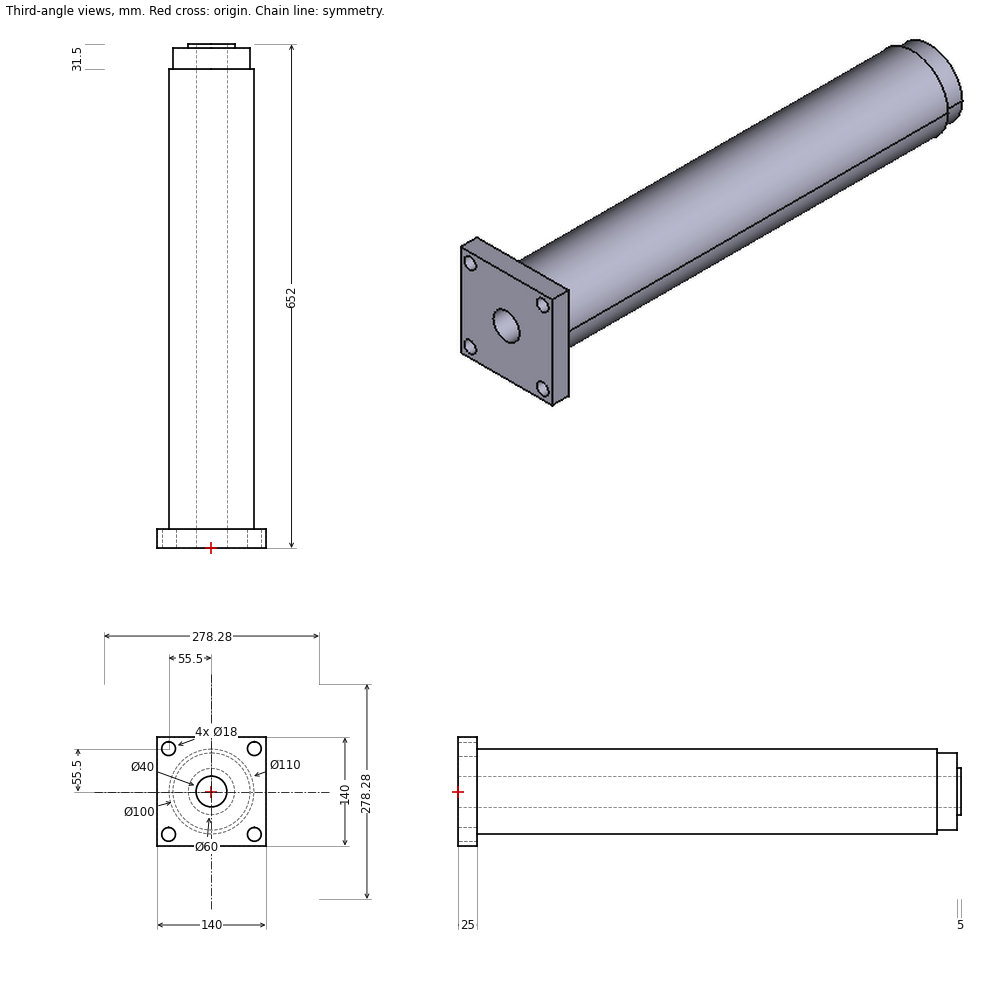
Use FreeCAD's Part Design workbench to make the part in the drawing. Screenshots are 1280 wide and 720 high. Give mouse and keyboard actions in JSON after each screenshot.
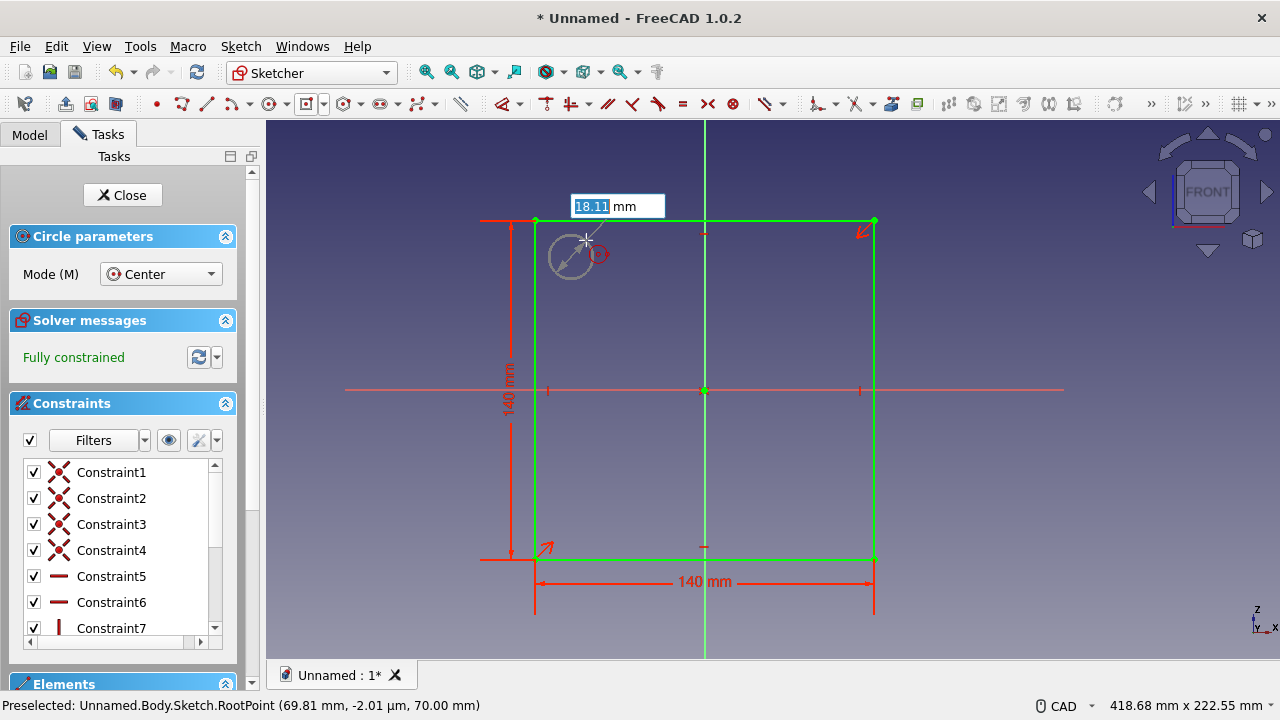
{"action": "type", "text": "18"}
{"action": "key", "text": "Return"}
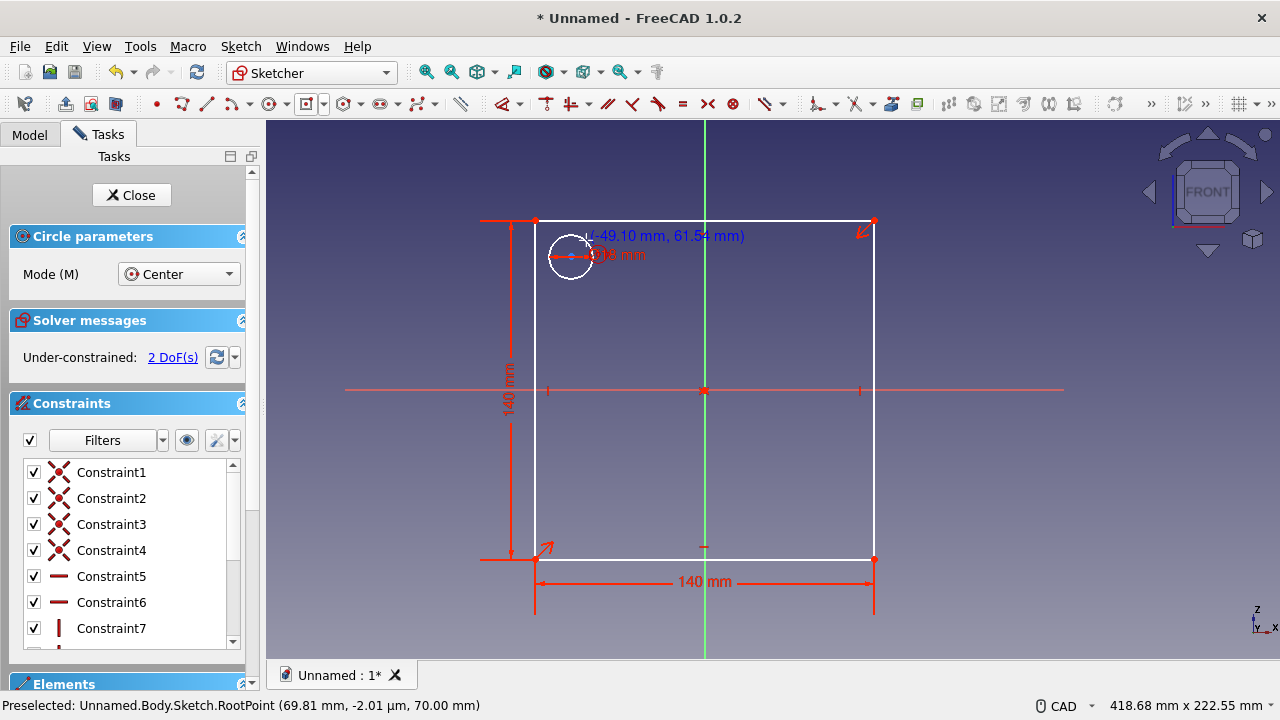
{"action": "left_click", "coordinate": [839, 256]}
{"action": "mouse_move", "coordinate": [855, 240]}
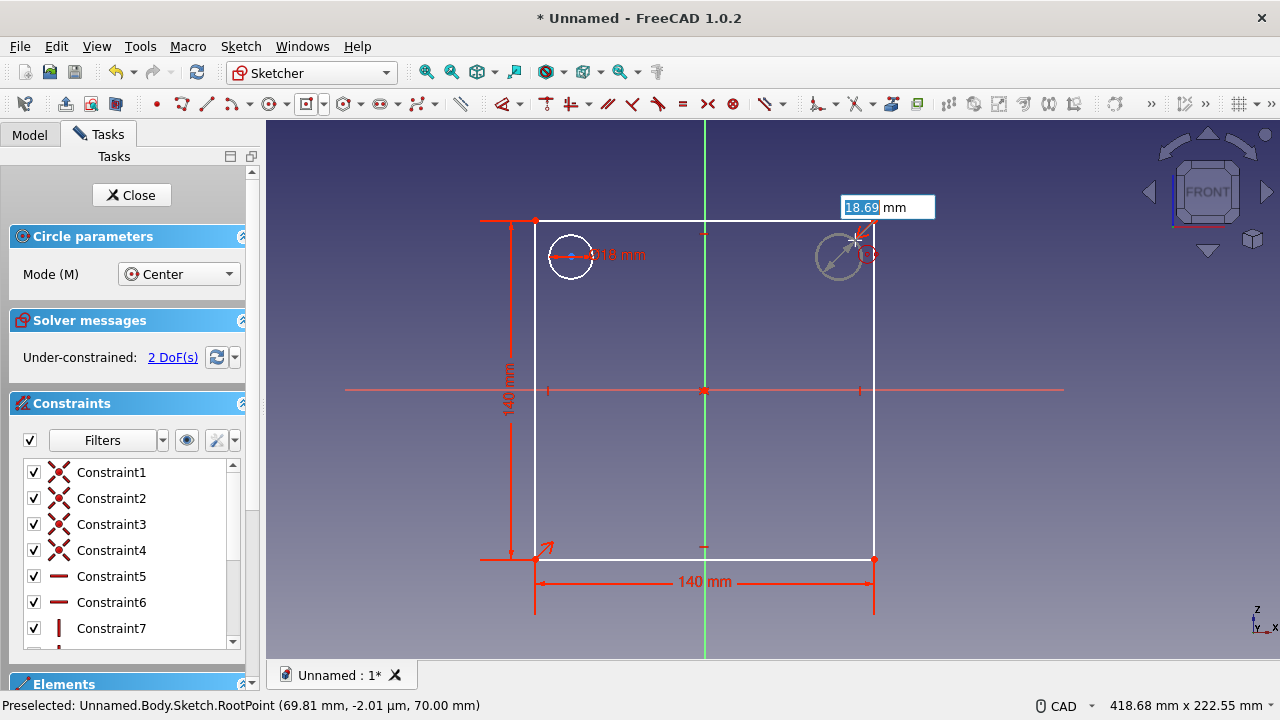
{"action": "type", "text": "18"}
{"action": "key", "text": "Return"}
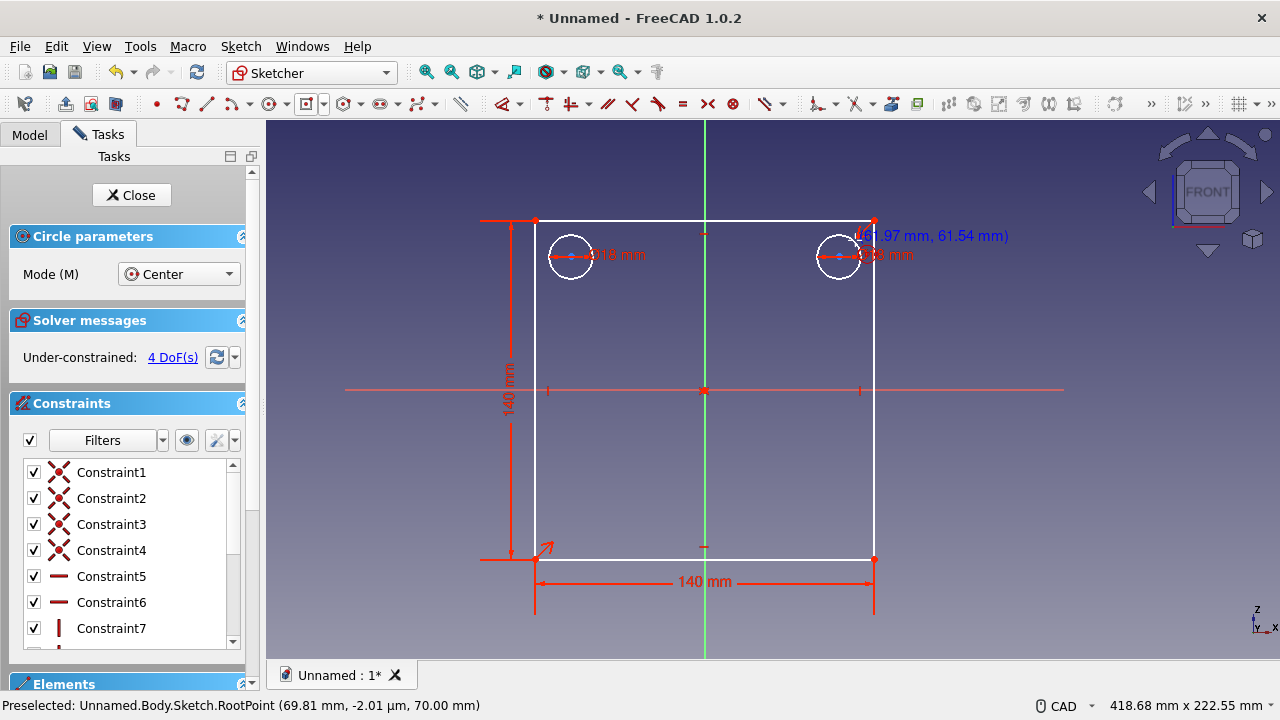
{"action": "left_click", "coordinate": [571, 524]}
{"action": "mouse_move", "coordinate": [586, 509]}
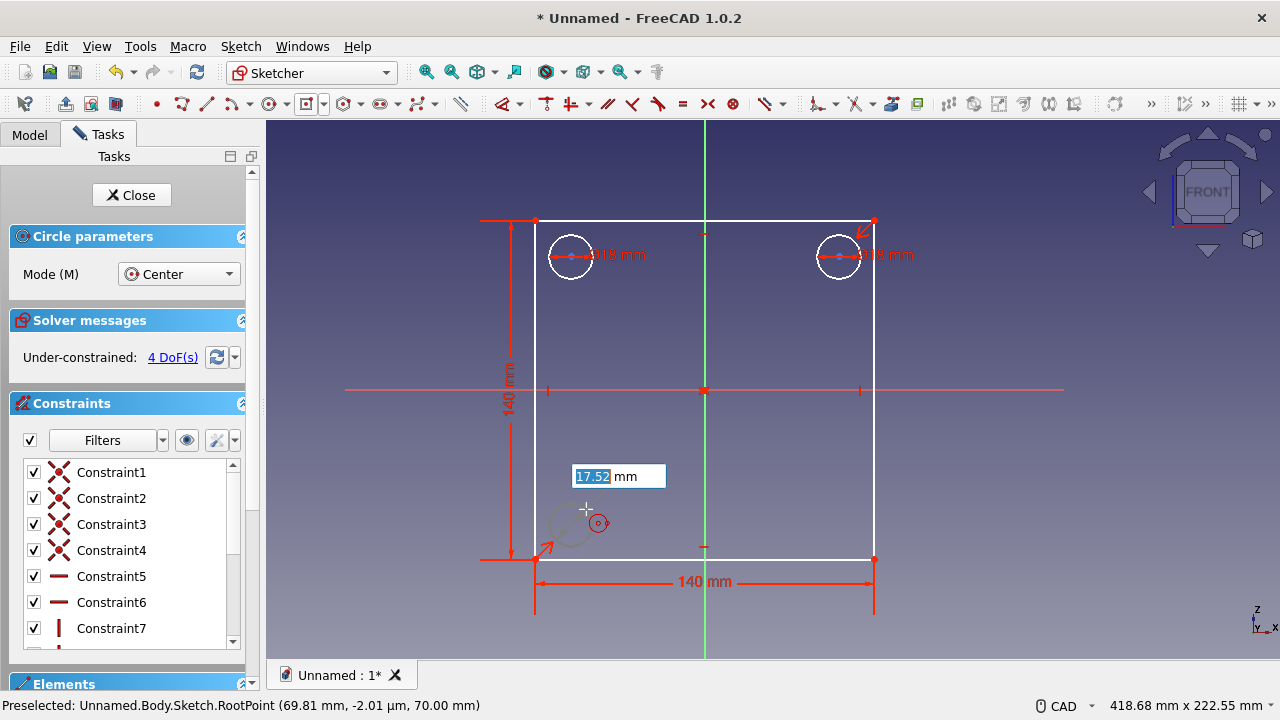
{"action": "type", "text": "18"}
{"action": "key", "text": "Return"}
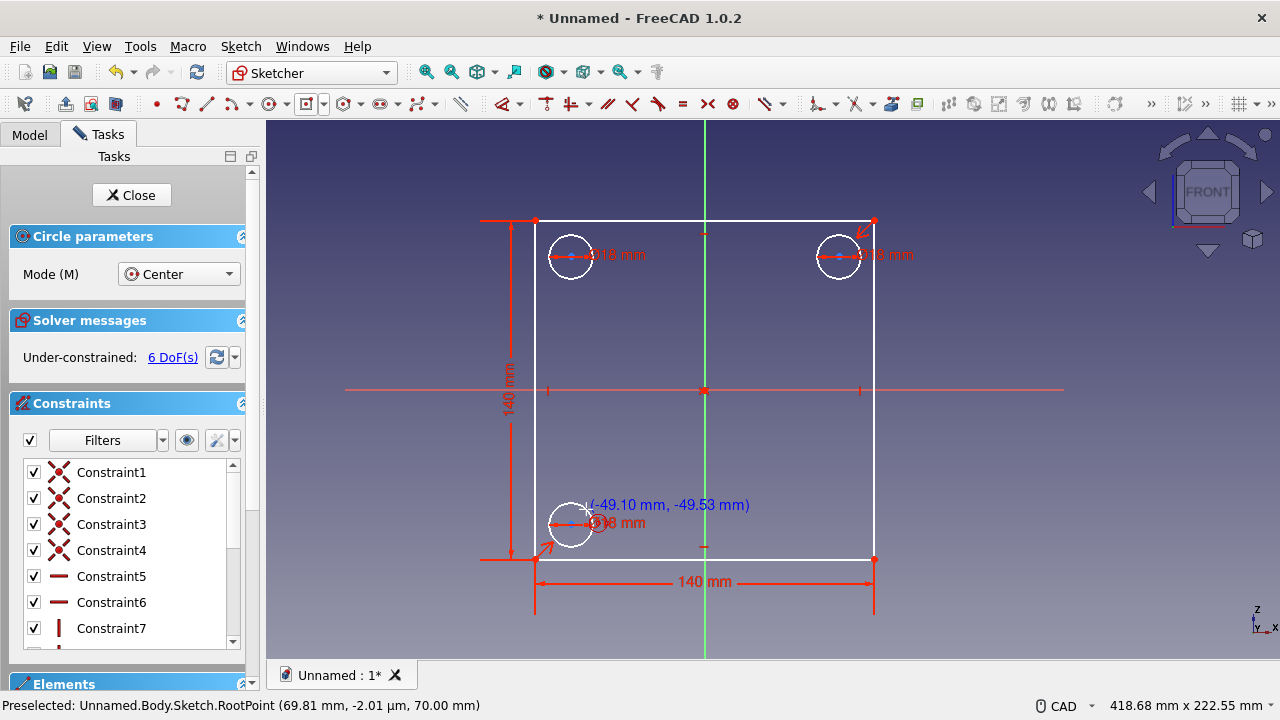
{"action": "left_click", "coordinate": [839, 524]}
{"action": "mouse_move", "coordinate": [855, 509]}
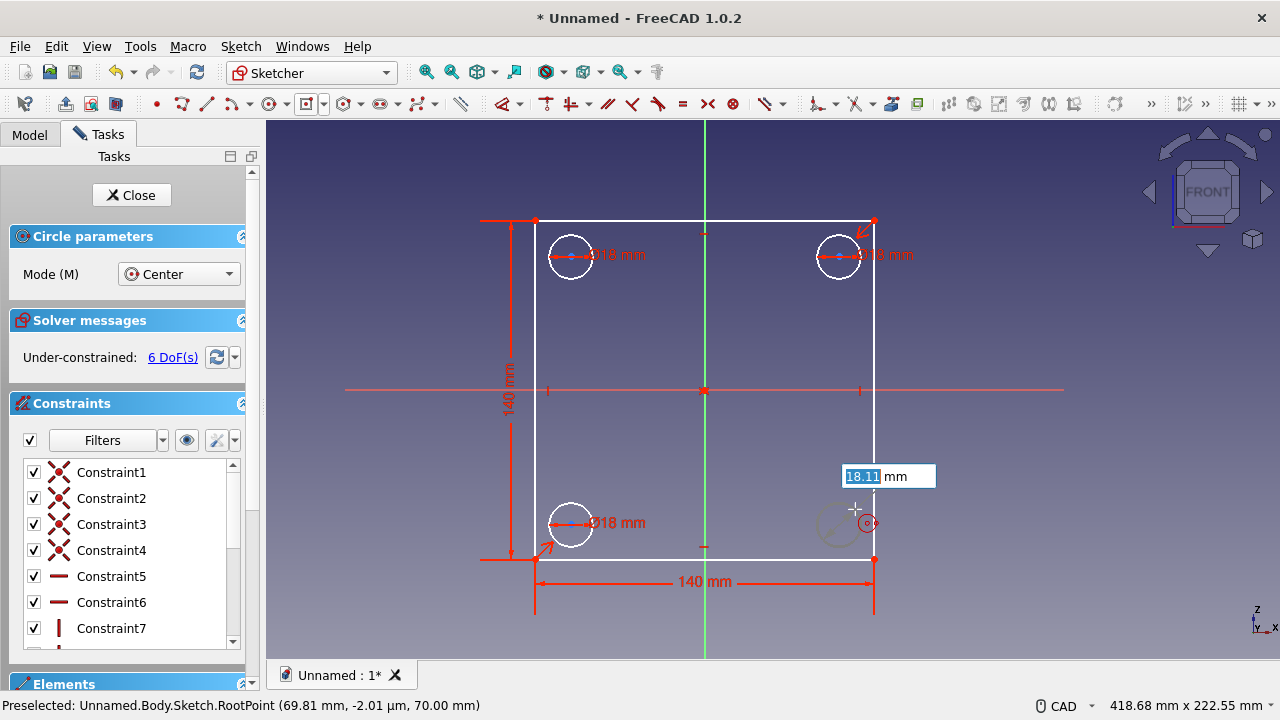
{"action": "type", "text": "18"}
{"action": "key", "text": "Return"}
{"action": "key", "text": "Escape"}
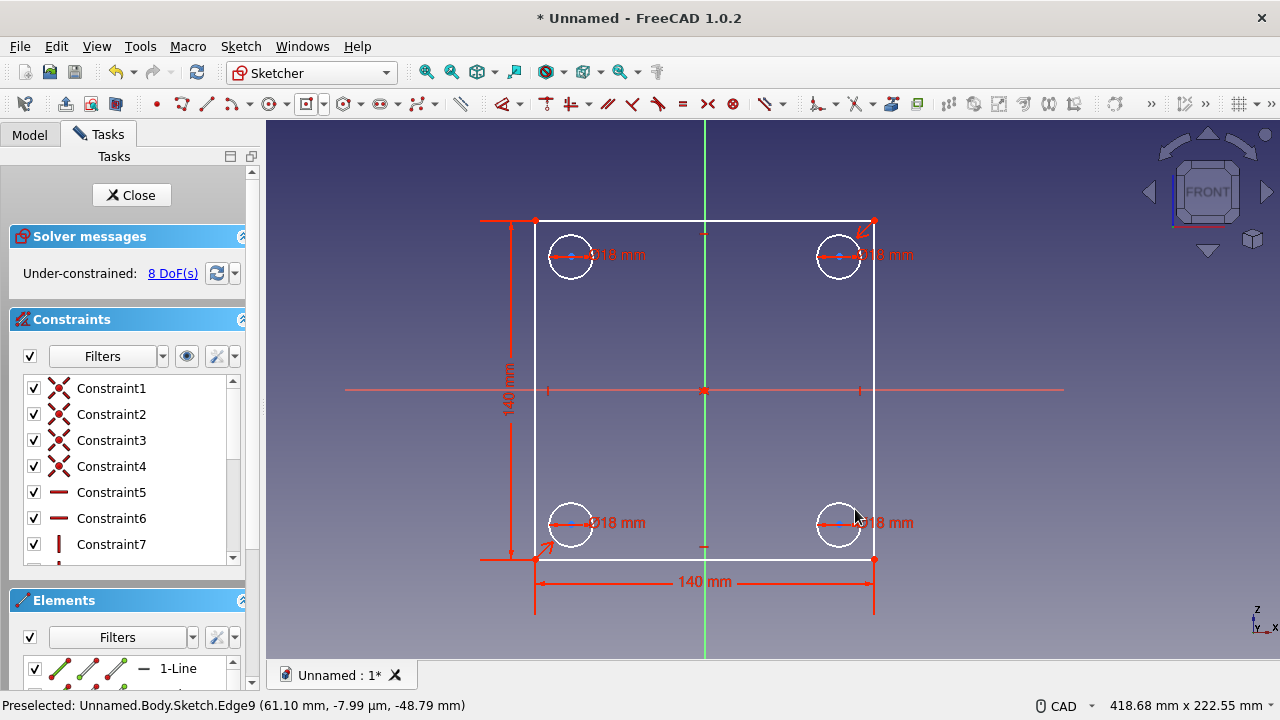
{"action": "left_click", "coordinate": [571, 257]}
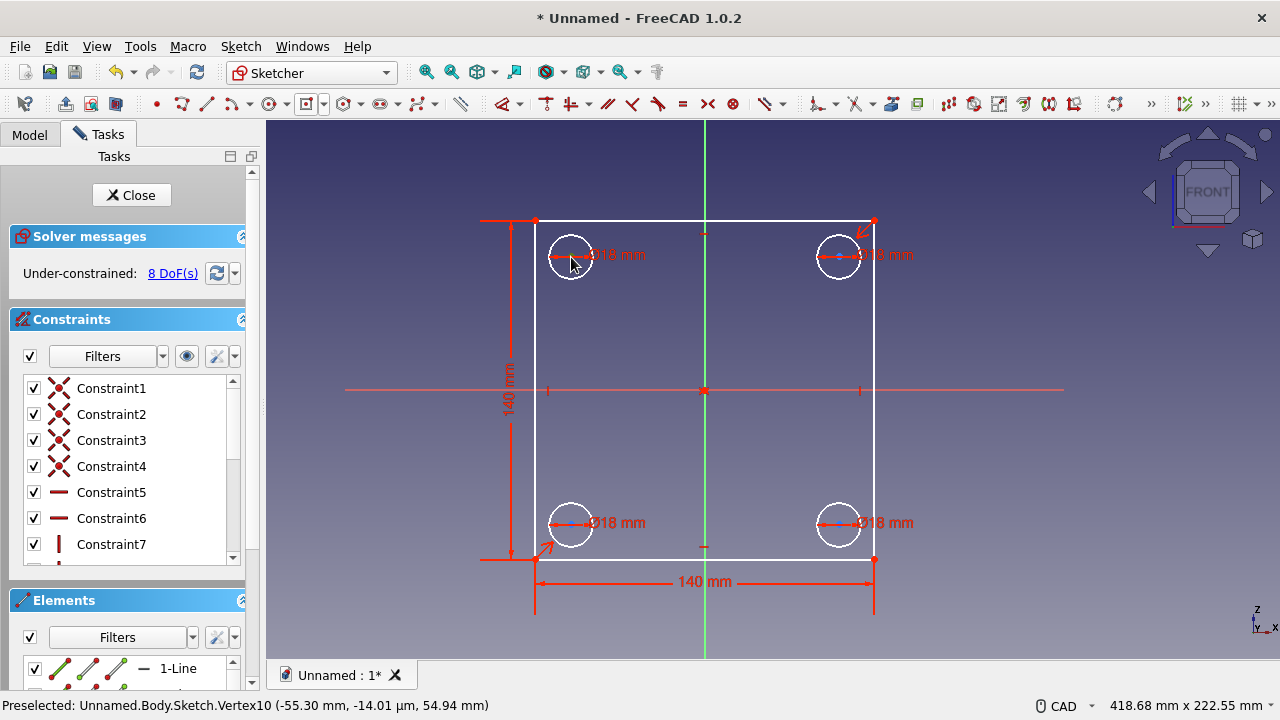
{"action": "left_click", "coordinate": [839, 257]}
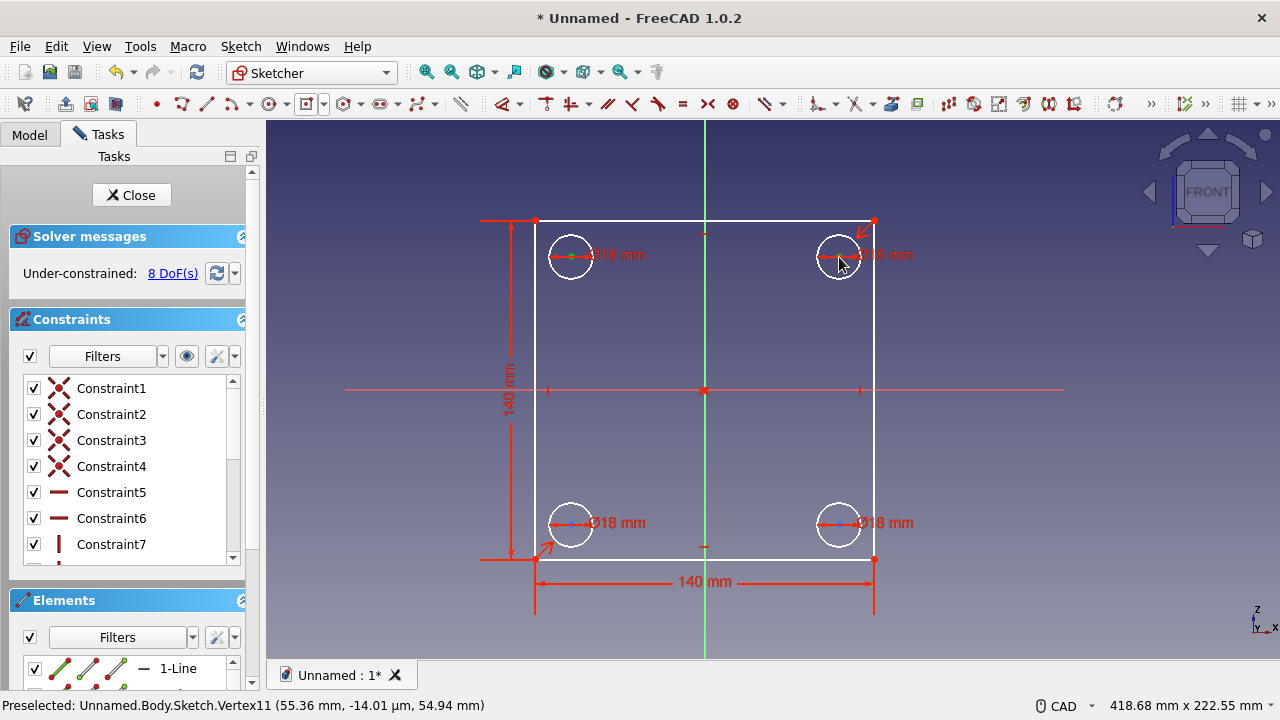
{"action": "left_click", "coordinate": [705, 596]}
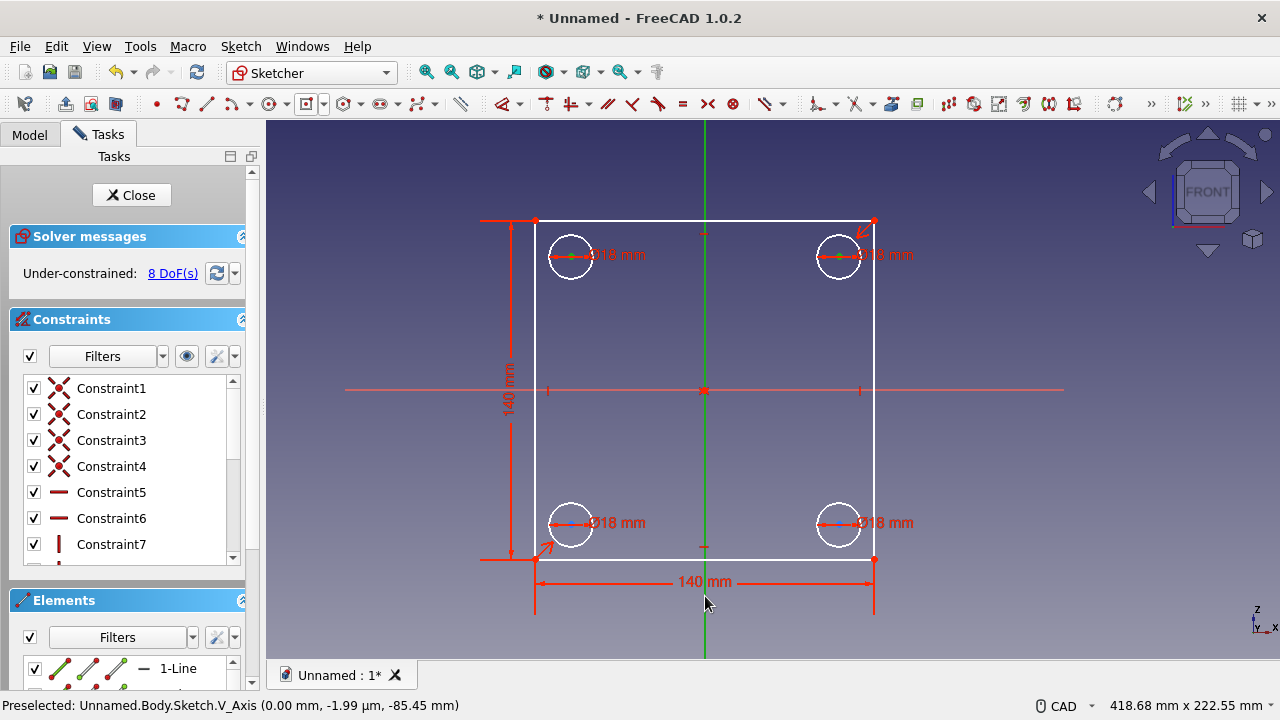
{"action": "left_click", "coordinate": [708, 104]}